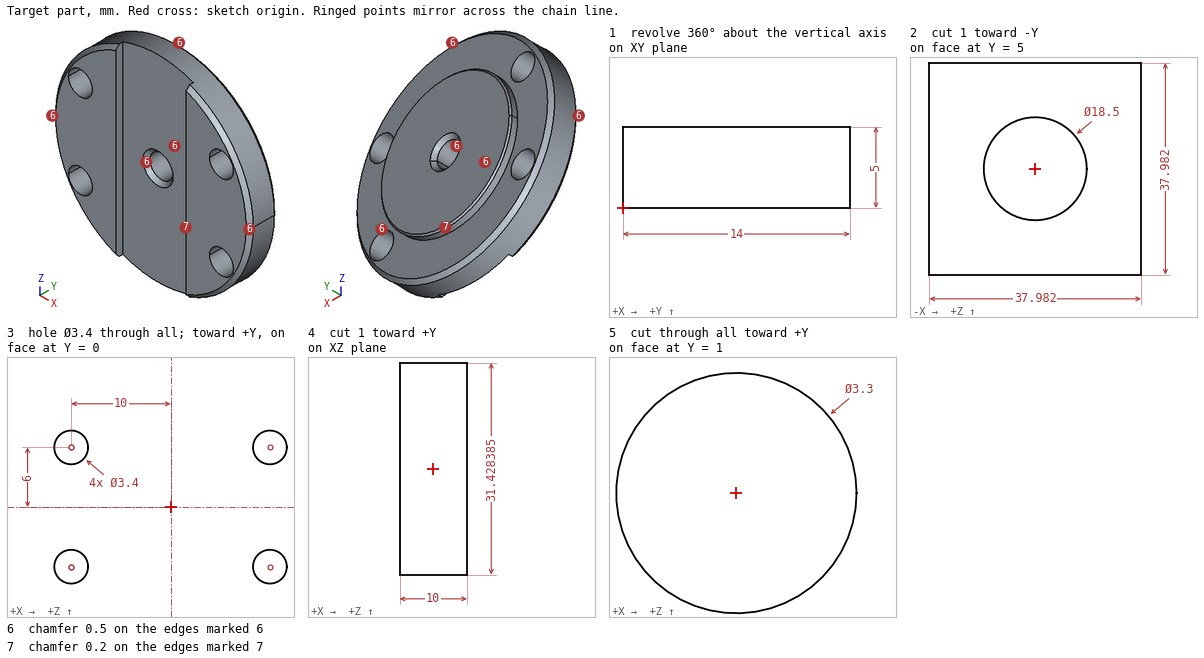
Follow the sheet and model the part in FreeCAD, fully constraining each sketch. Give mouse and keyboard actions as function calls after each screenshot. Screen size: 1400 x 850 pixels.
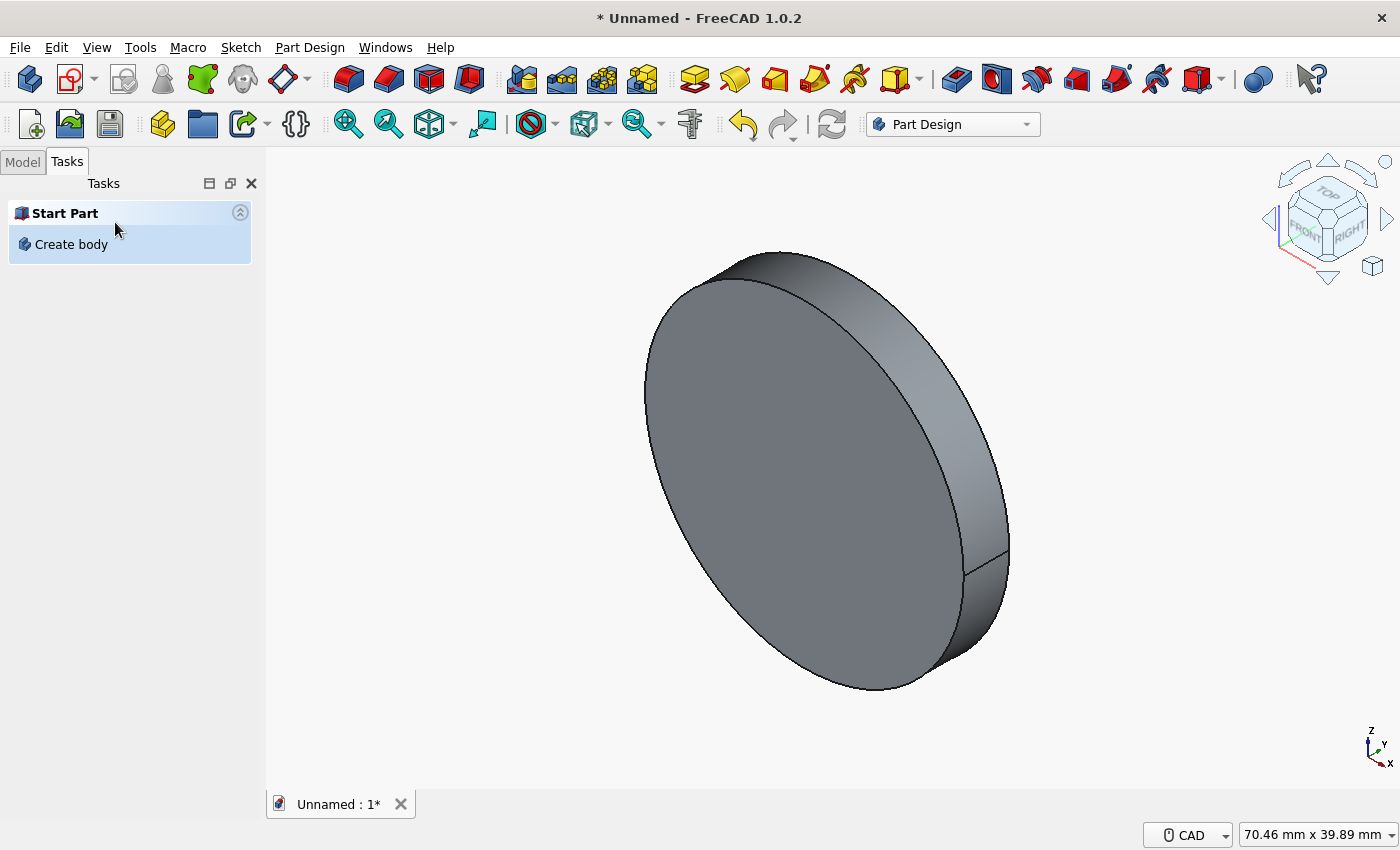
click(804, 483)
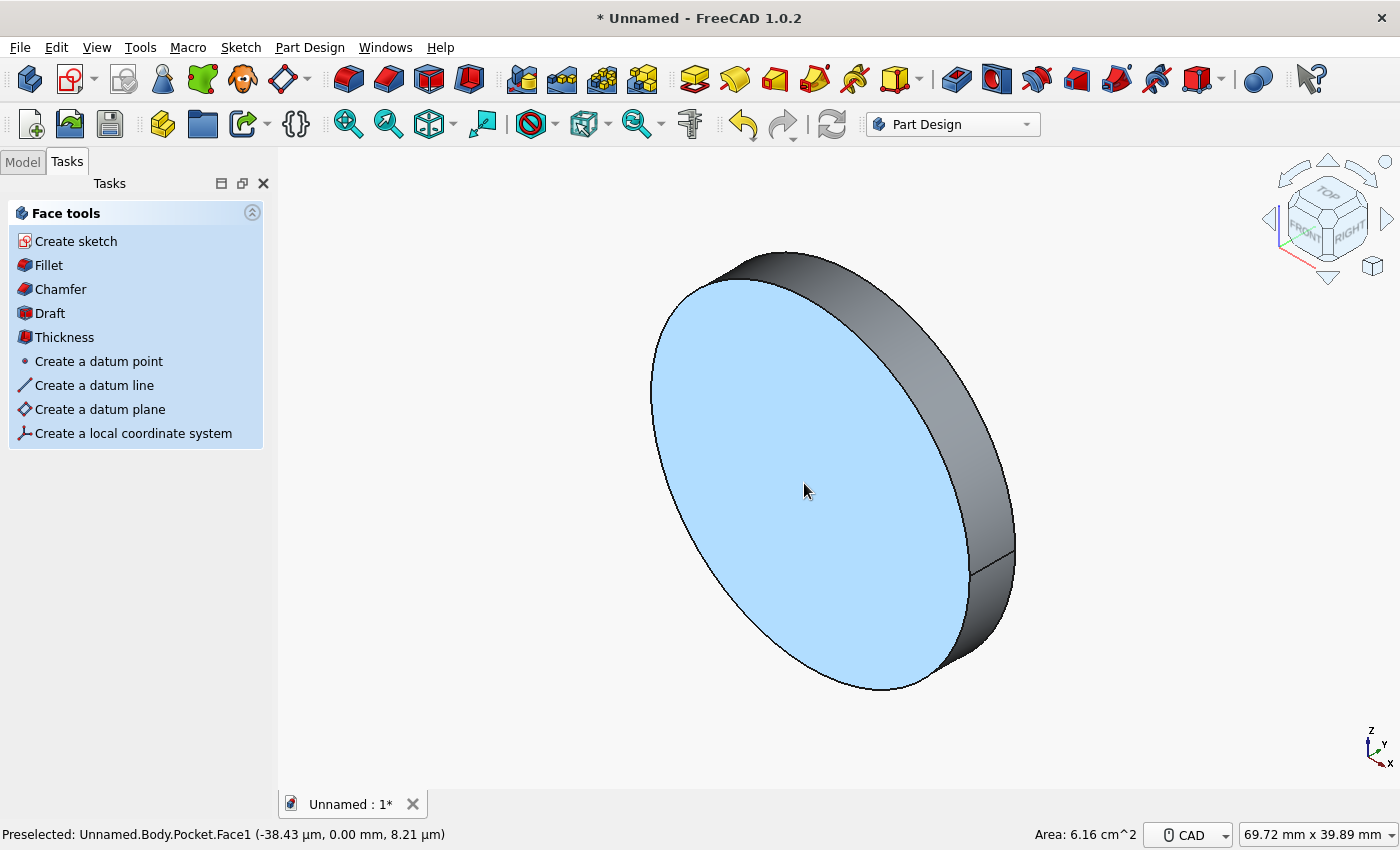
click(70, 80)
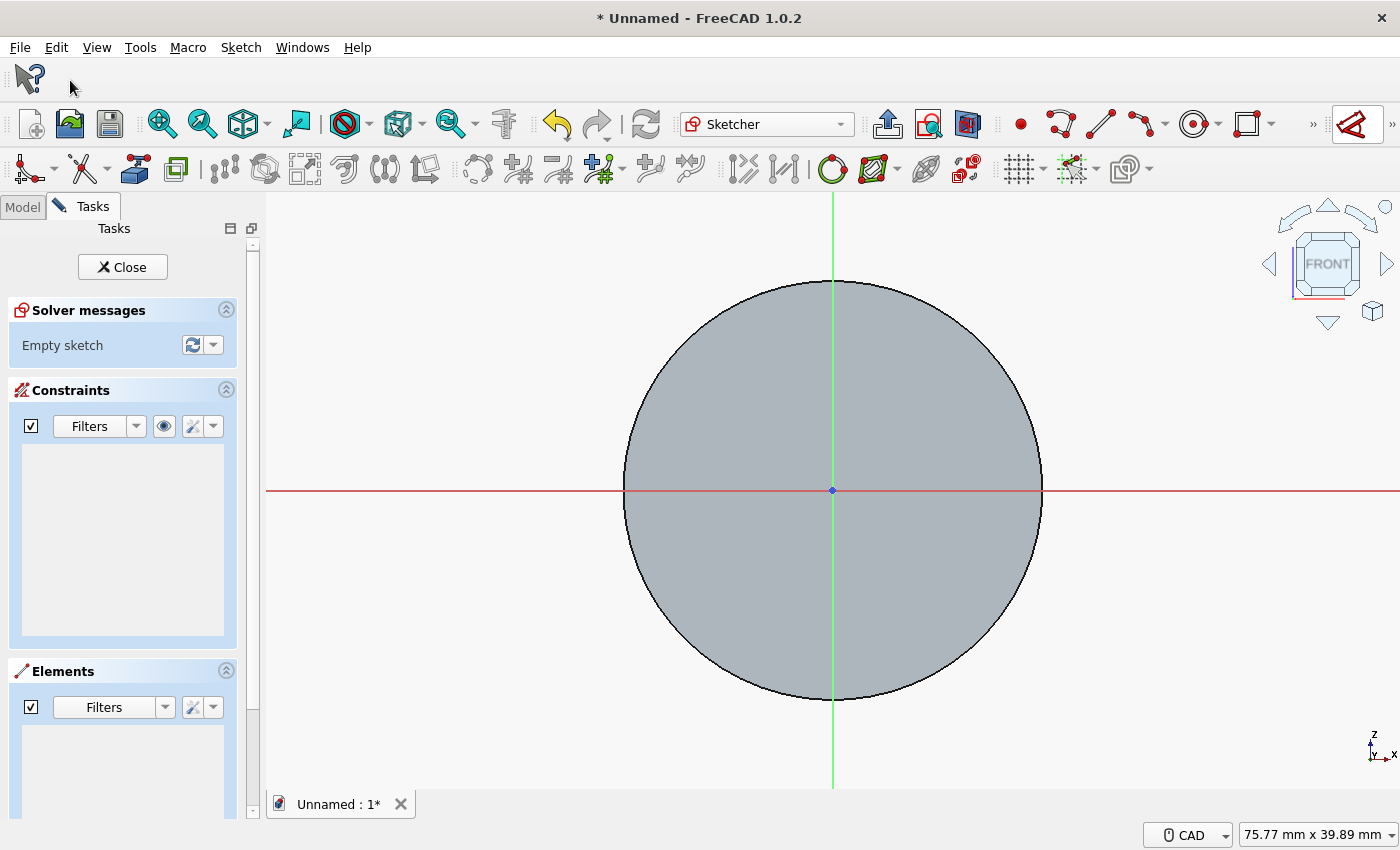
scroll(916, 491, up, 3)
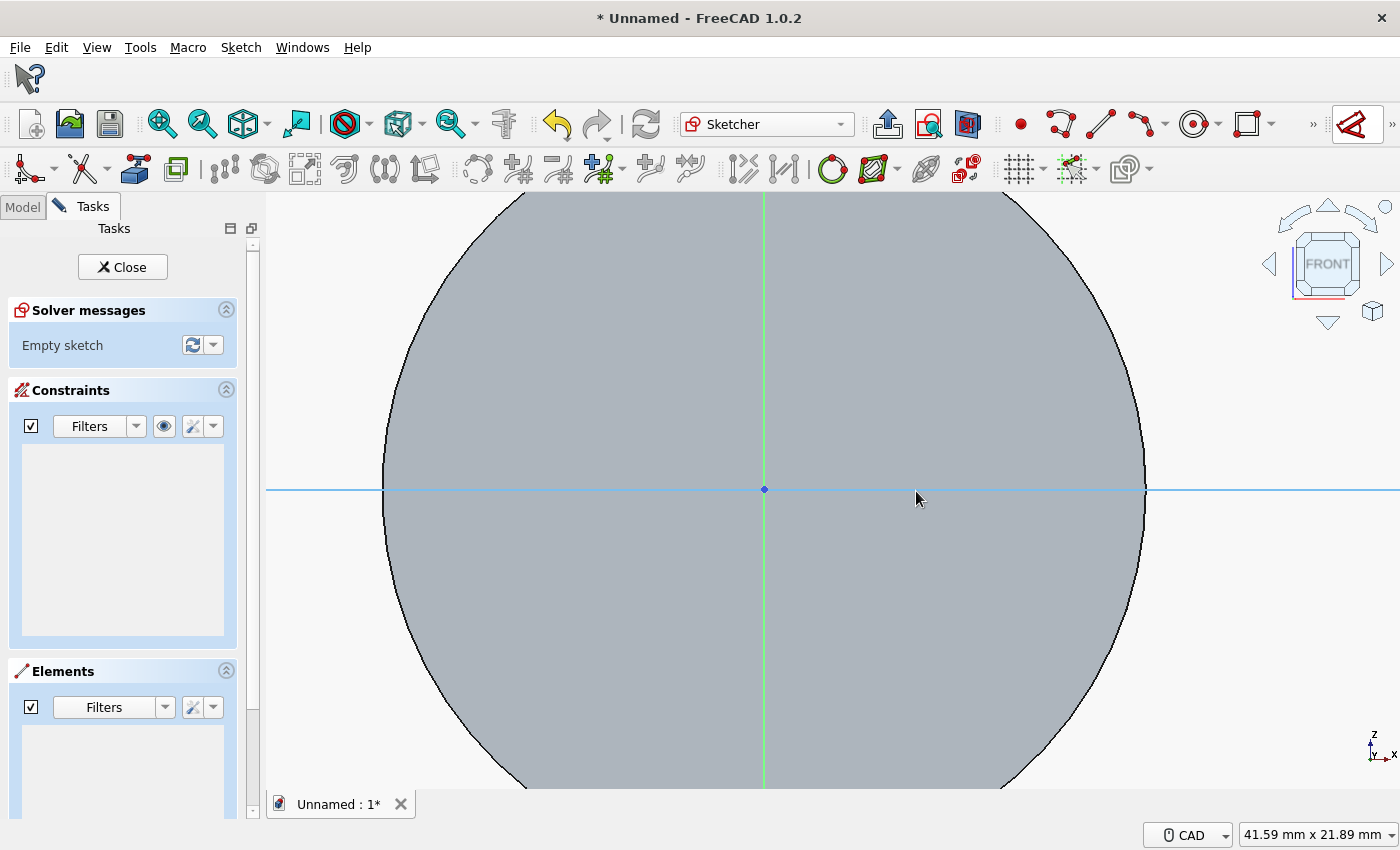
key(g)
key(c)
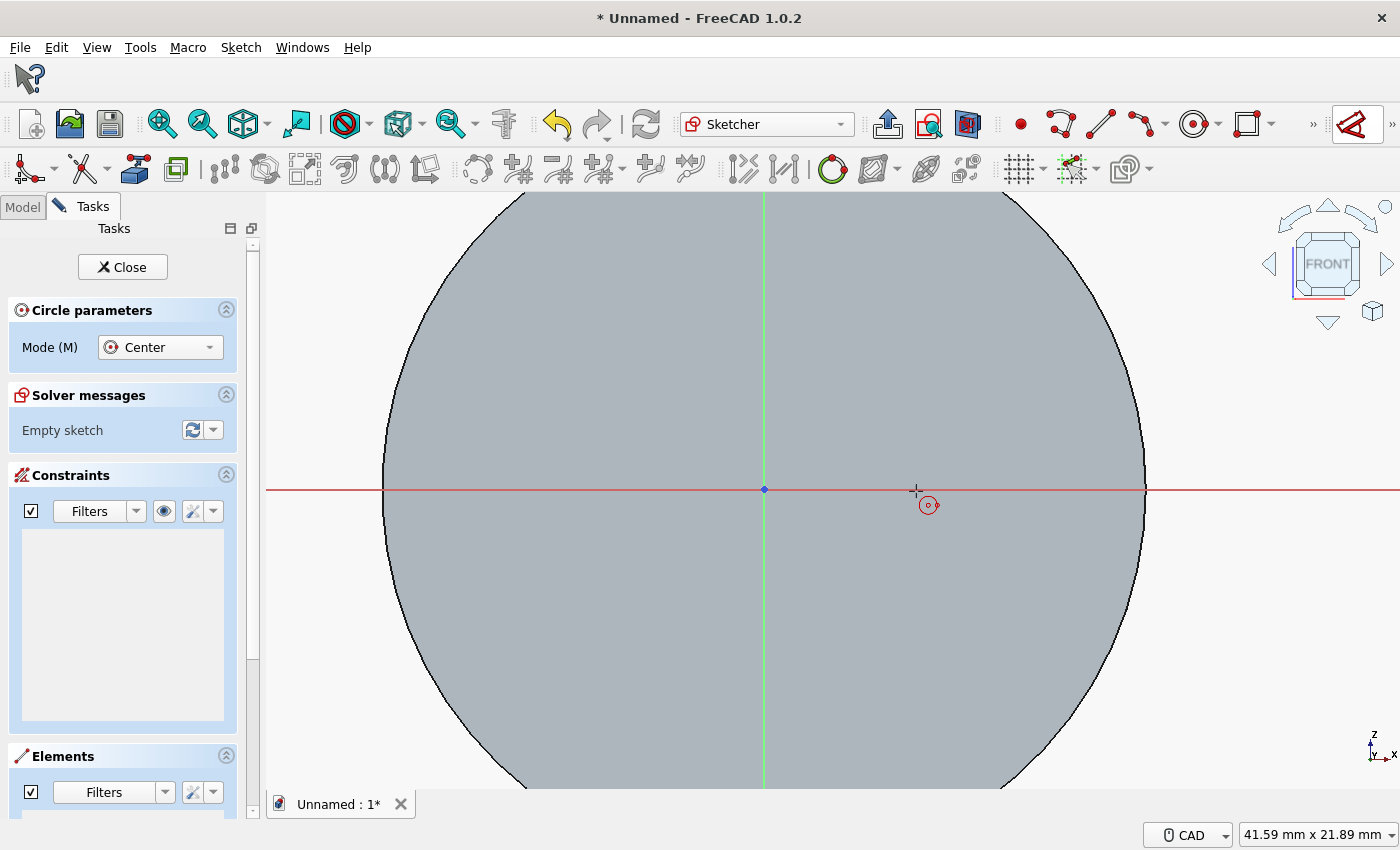
click(491, 326)
move(524, 293)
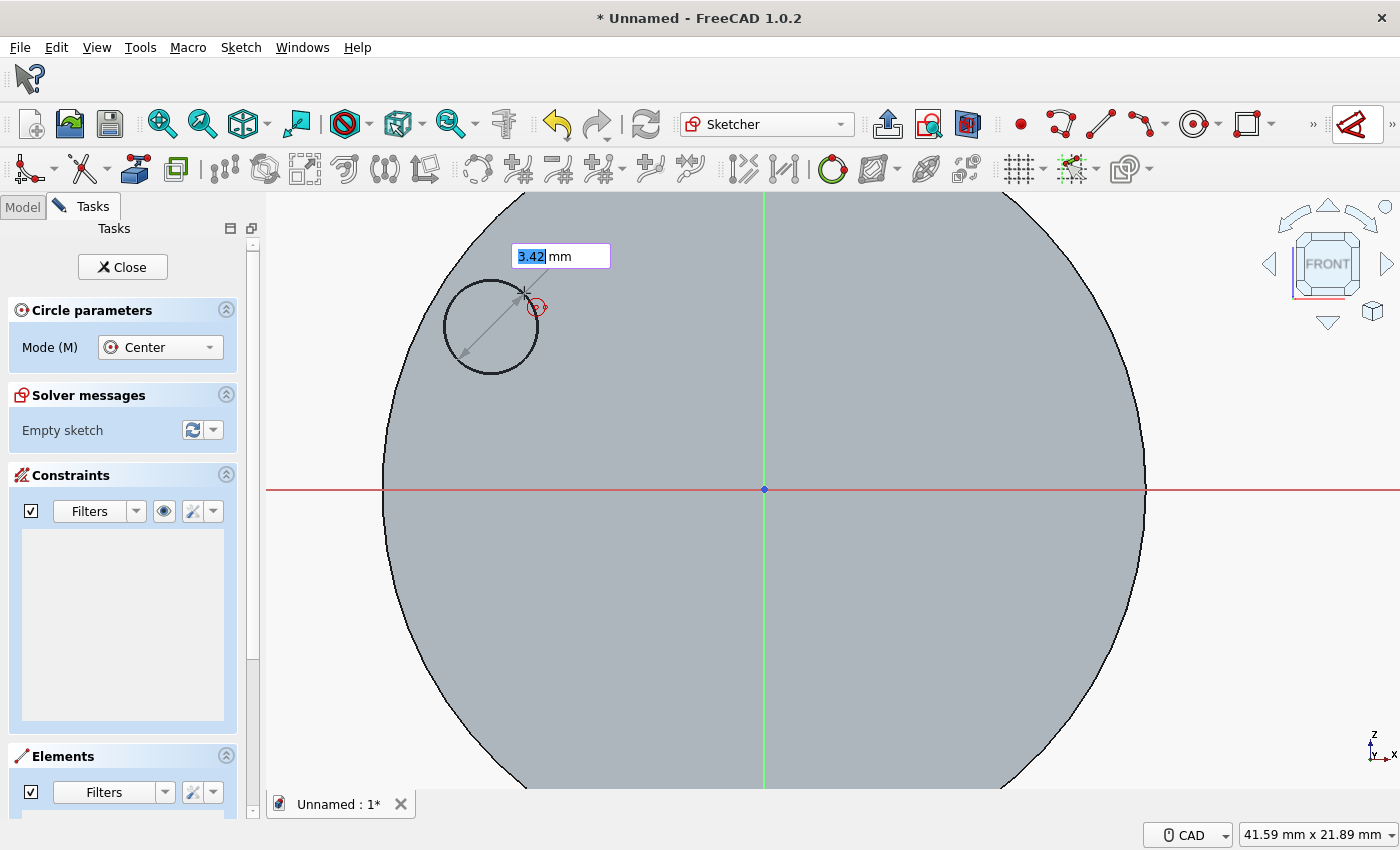
text(3.4)
key(Return)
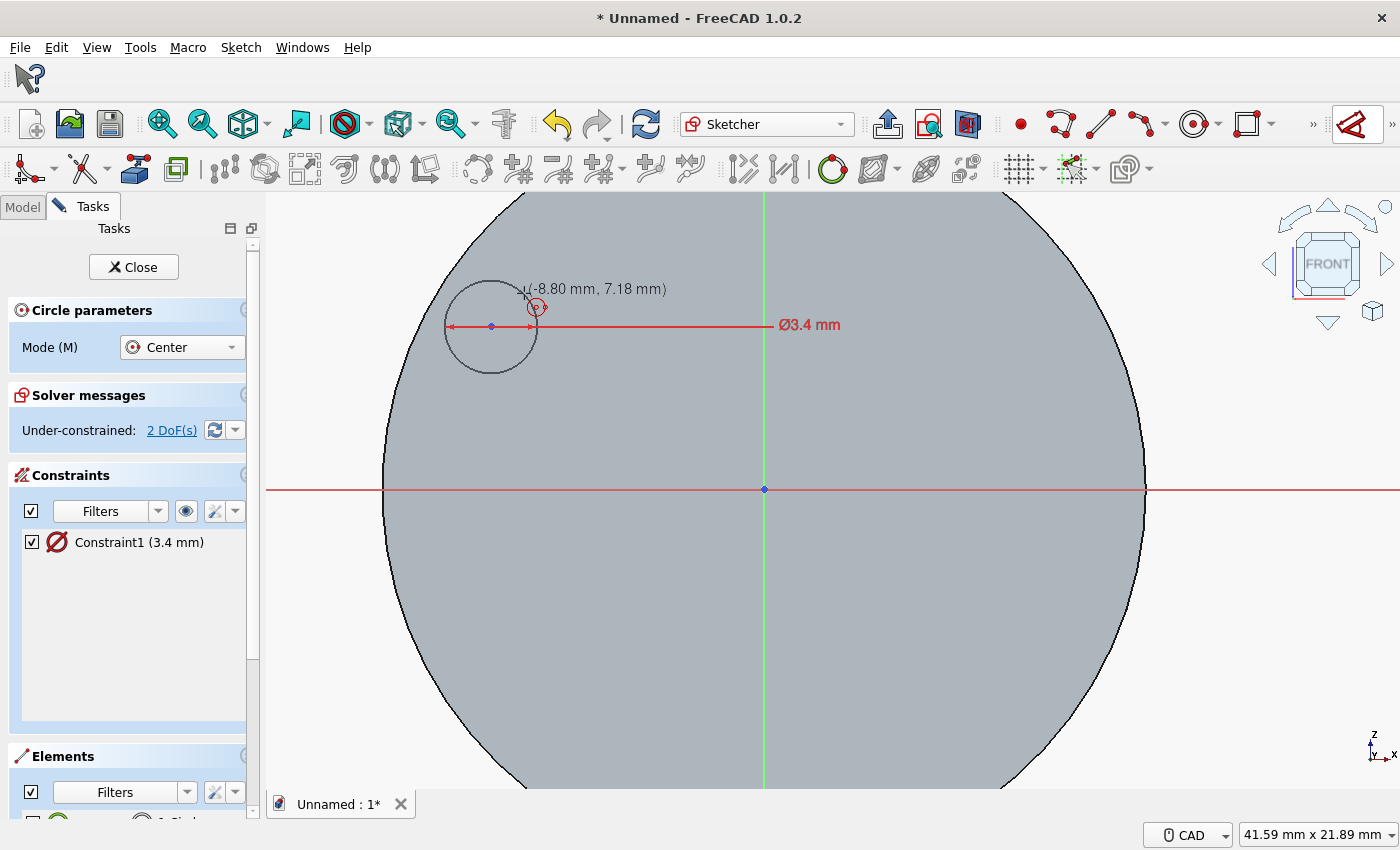
click(491, 653)
move(524, 621)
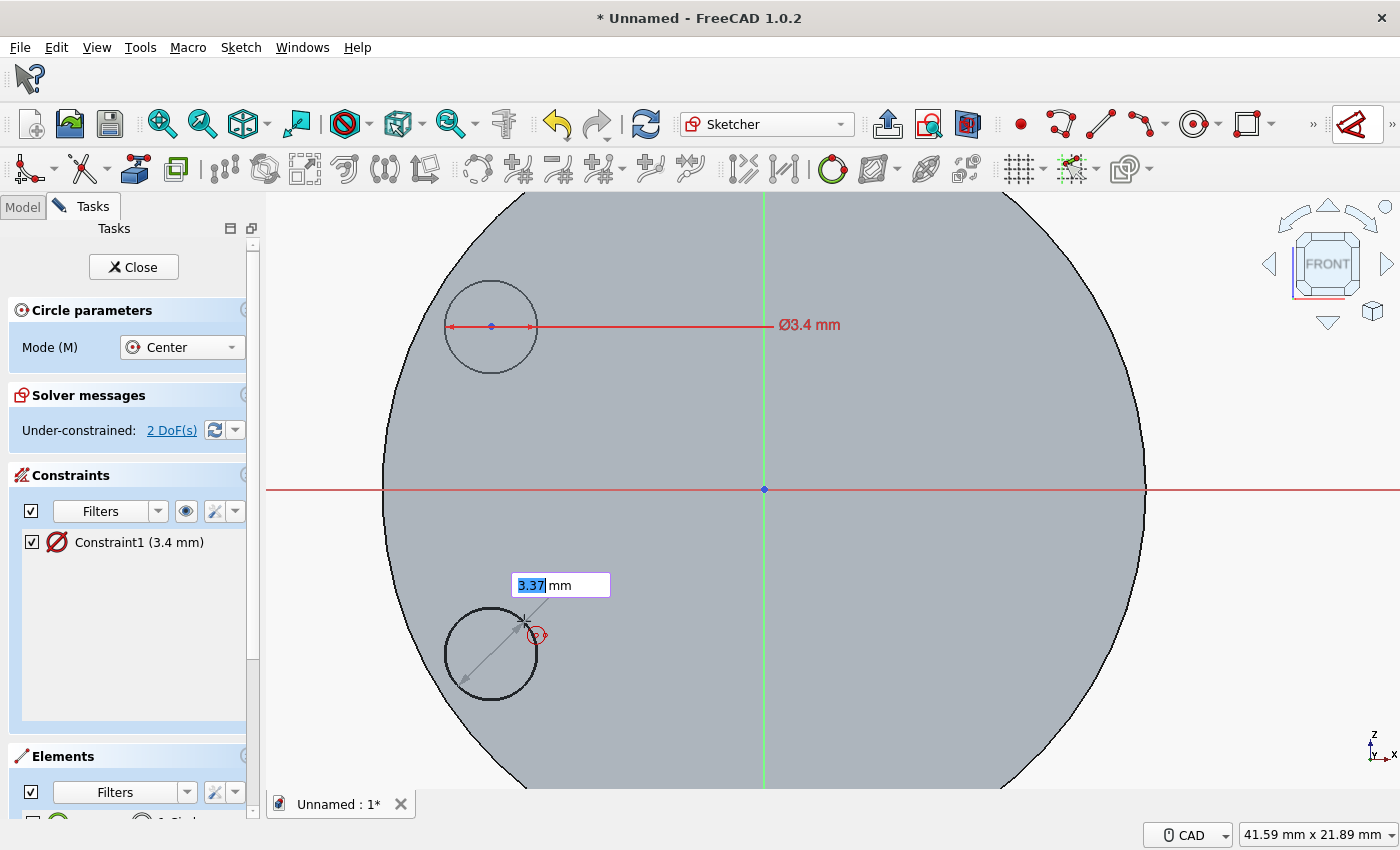
text(3.4)
key(Return)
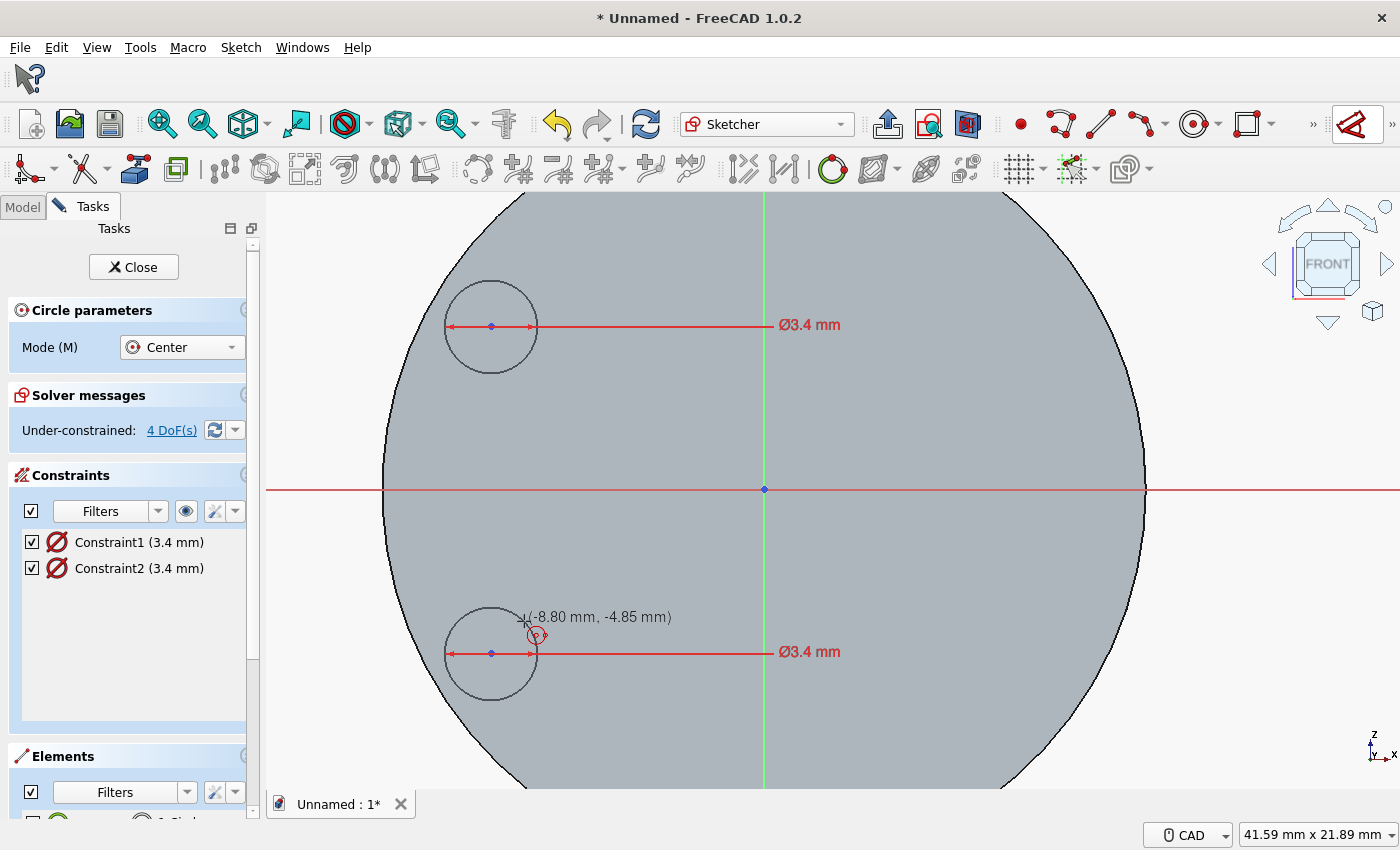
click(1037, 326)
move(1069, 293)